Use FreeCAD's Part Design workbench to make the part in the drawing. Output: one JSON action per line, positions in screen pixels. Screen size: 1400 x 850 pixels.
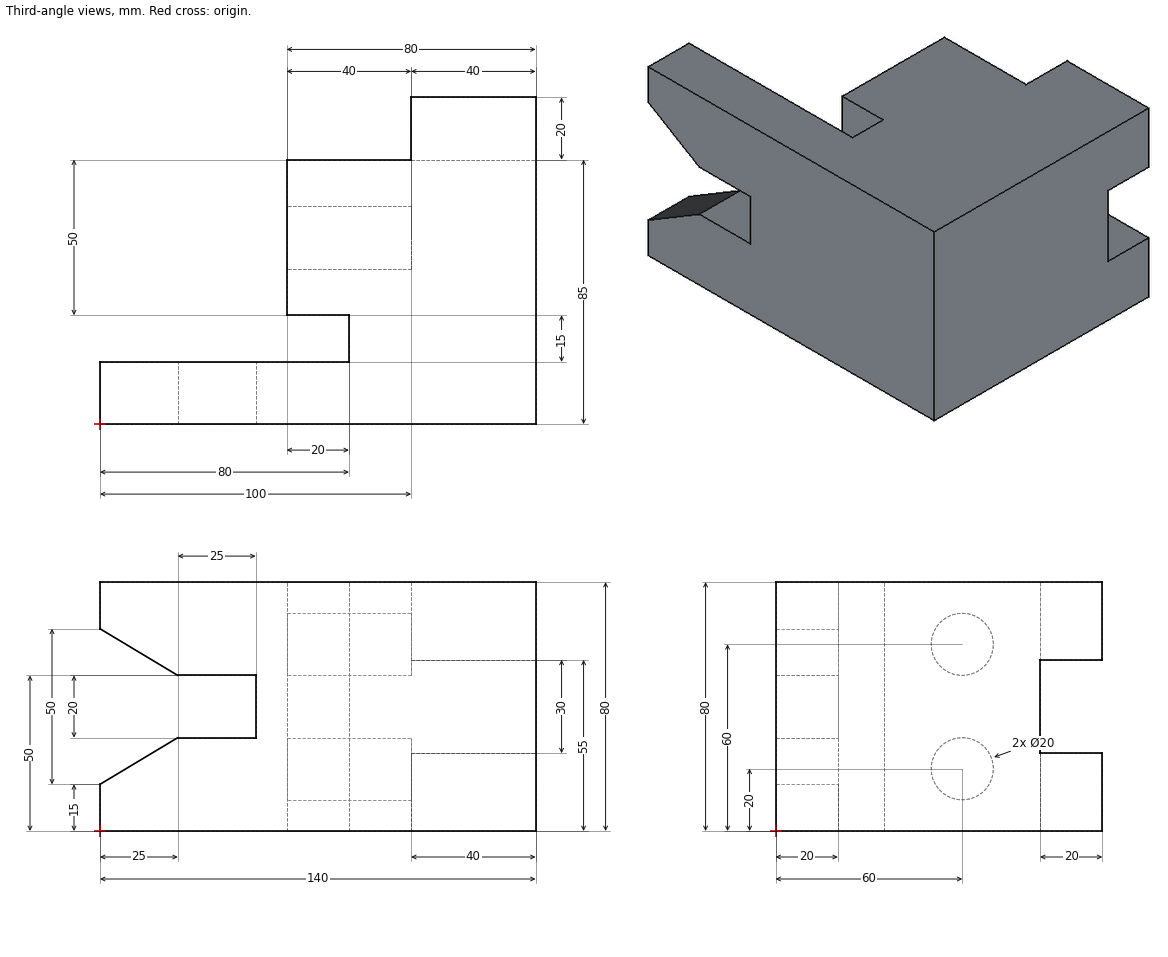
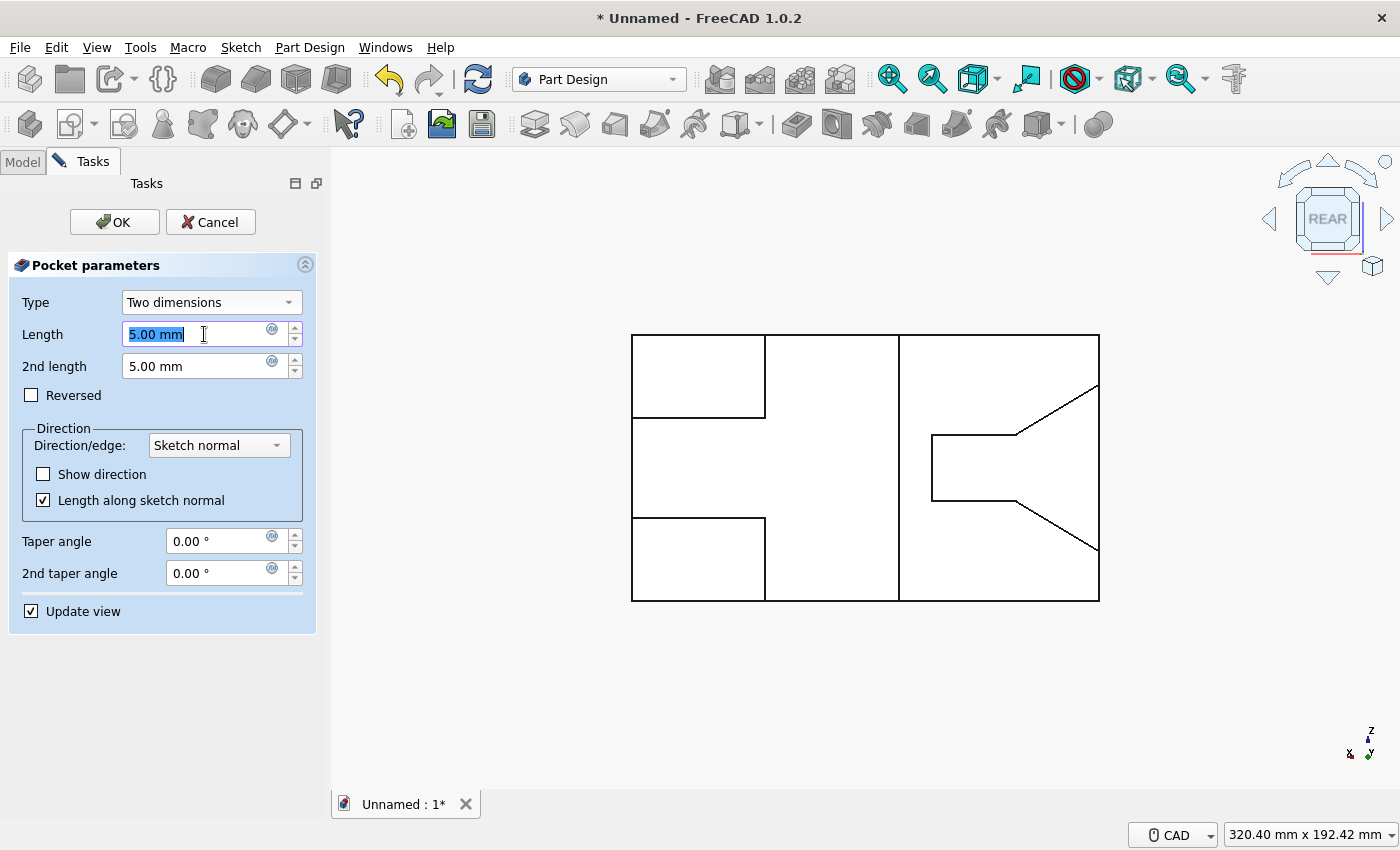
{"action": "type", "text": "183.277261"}
{"action": "key", "text": "Tab"}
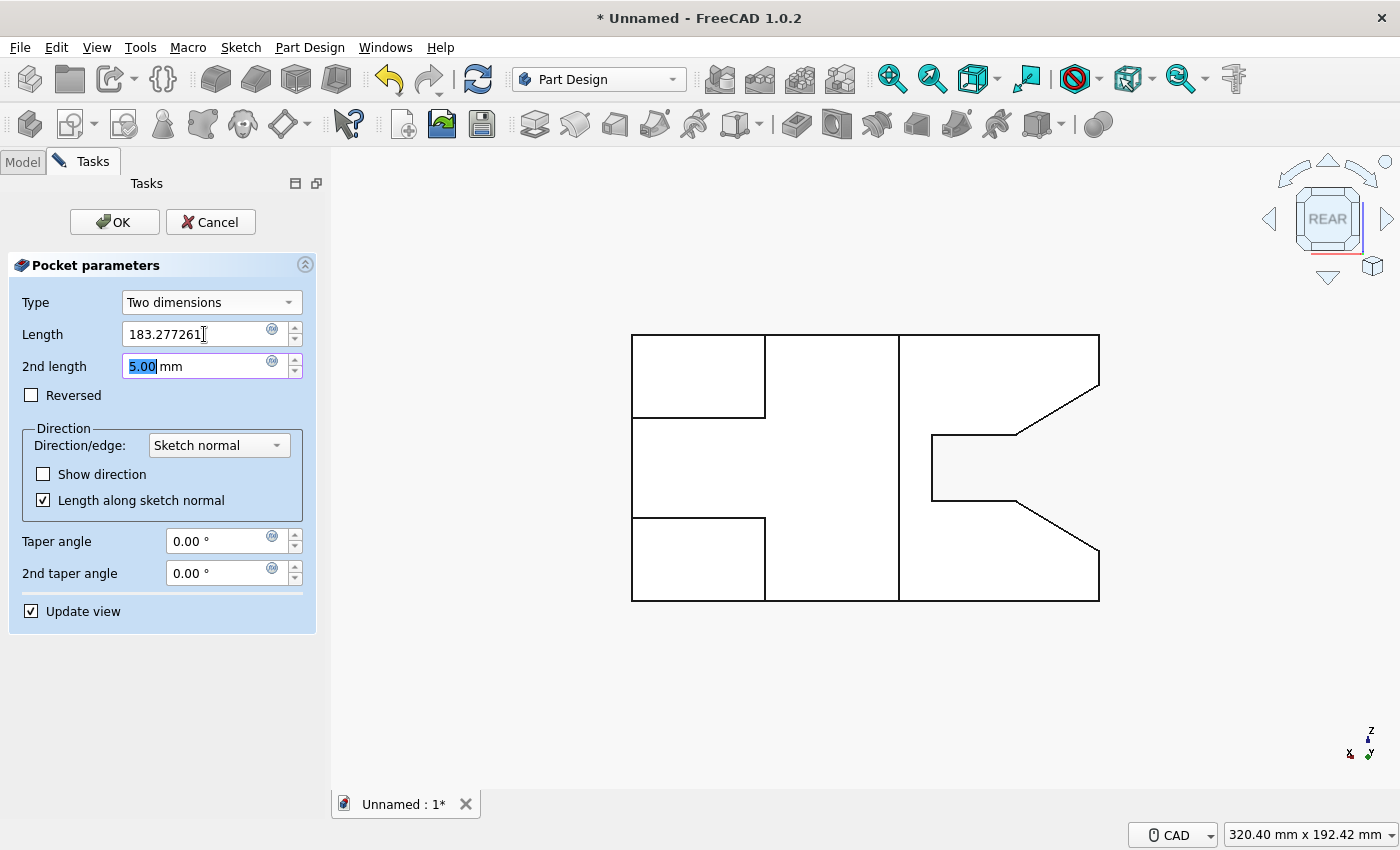
{"action": "type", "text": "20"}
{"action": "key", "text": "Tab"}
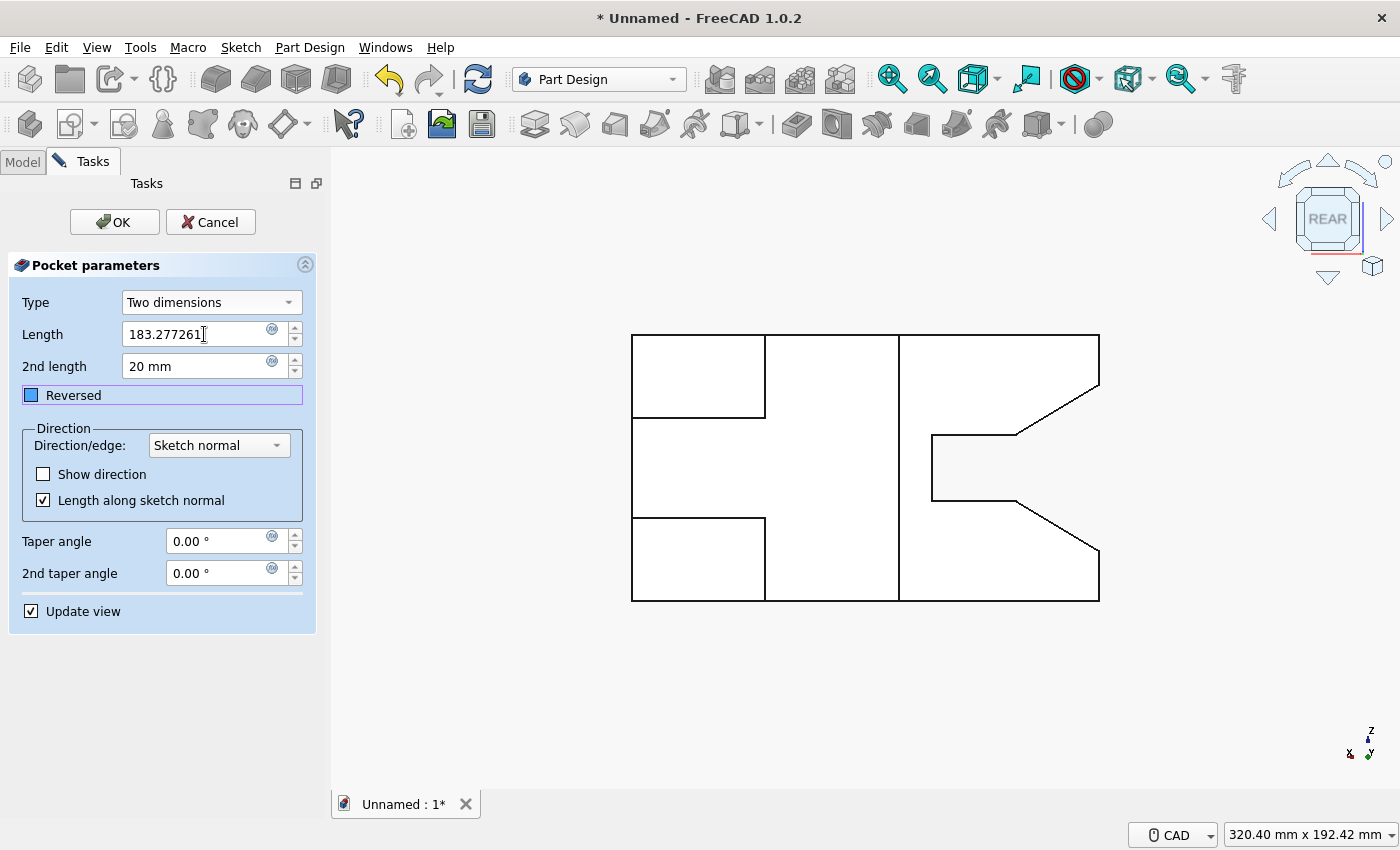
{"action": "left_click", "coordinate": [30, 395]}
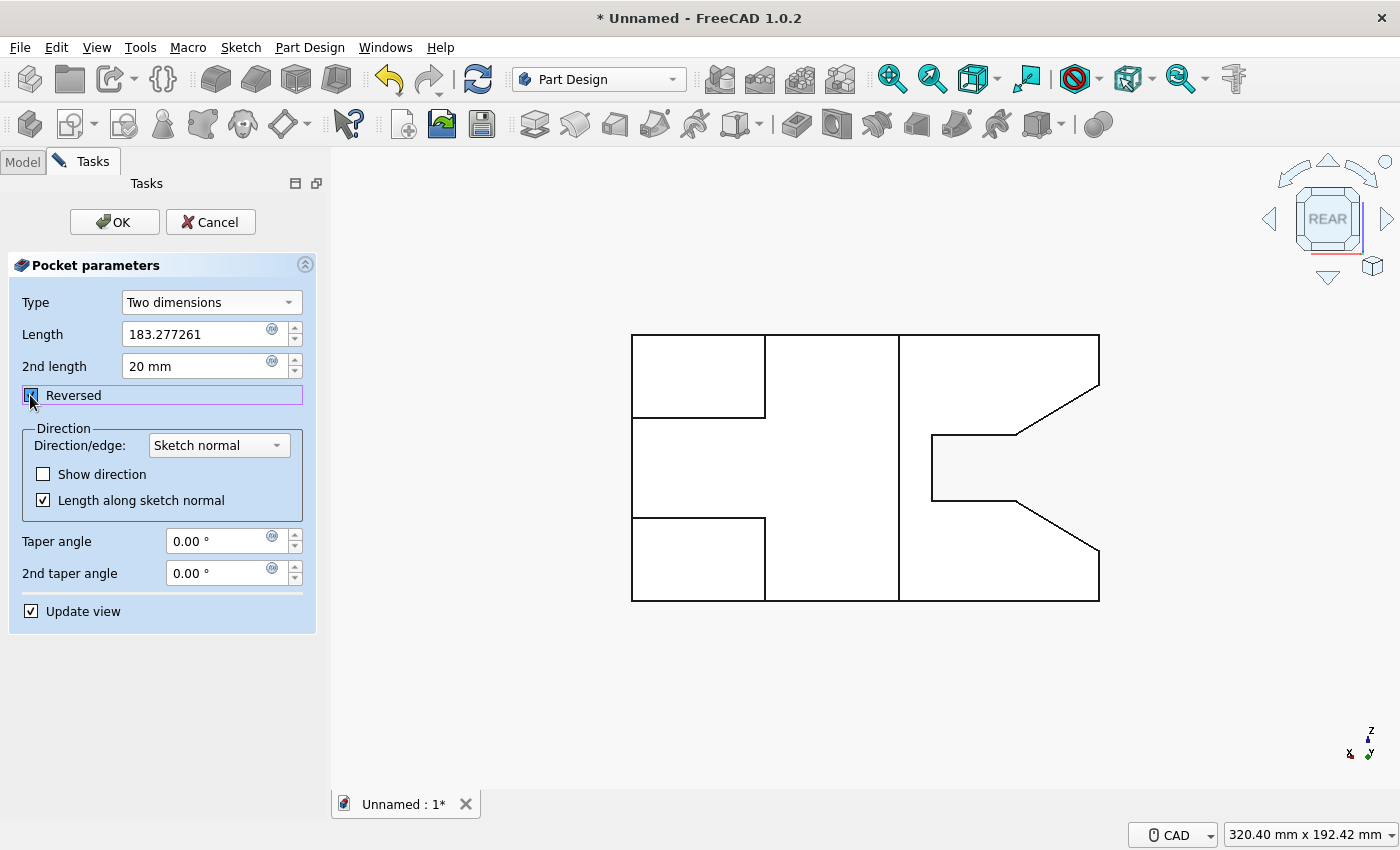
{"action": "left_click", "coordinate": [115, 222]}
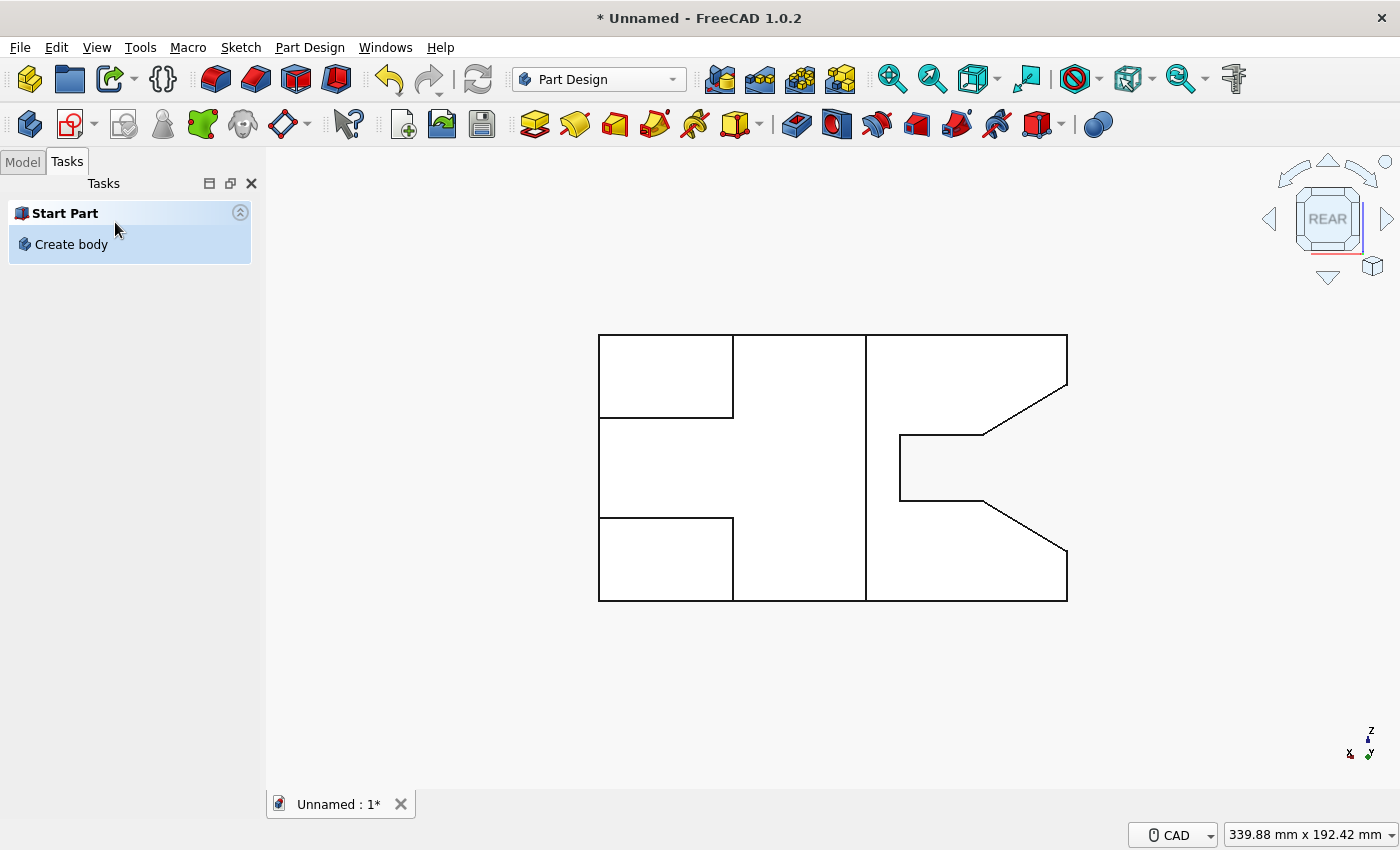
{"action": "key", "text": "v f"}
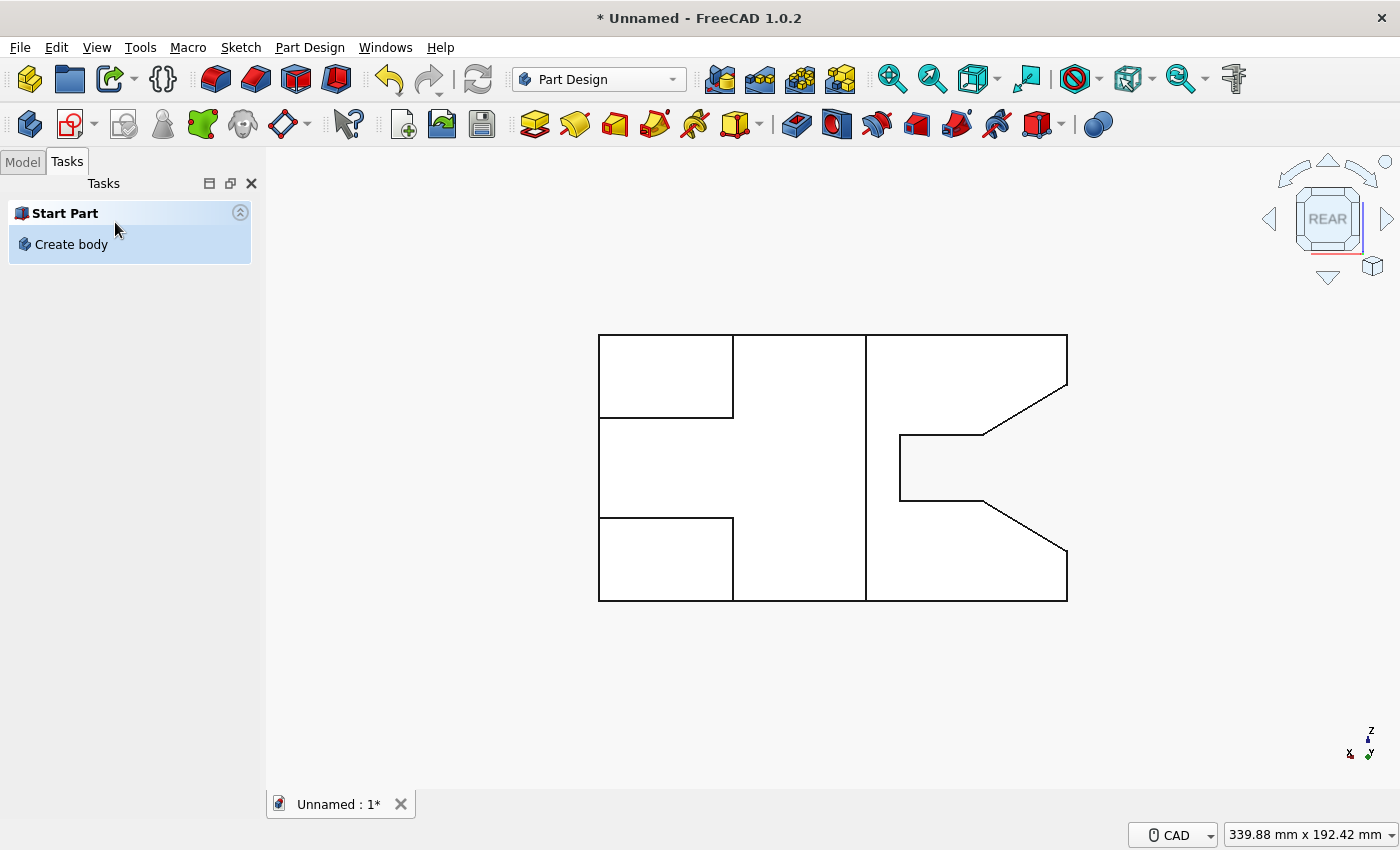
{"action": "key", "text": "6"}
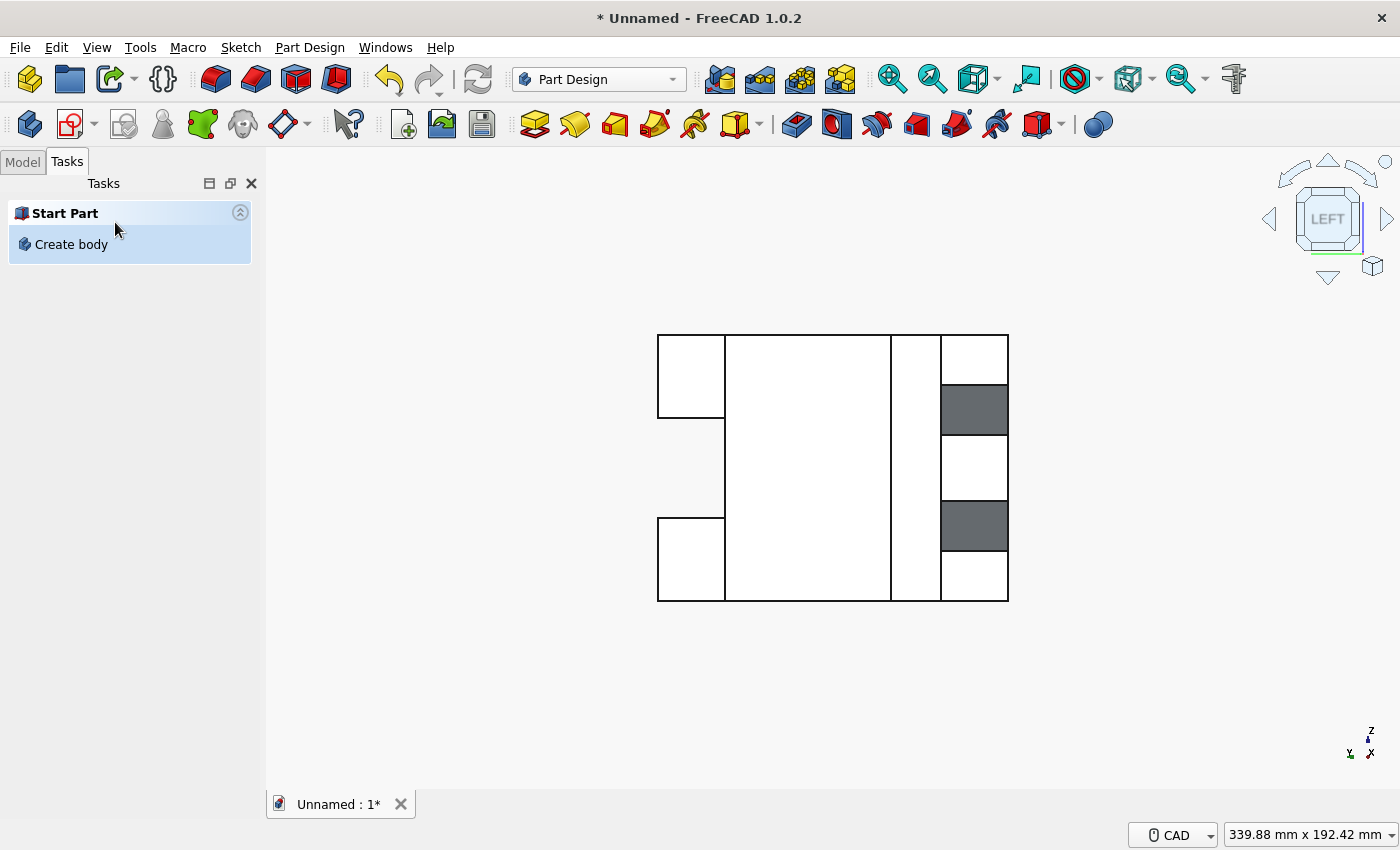
{"action": "key", "text": "v f"}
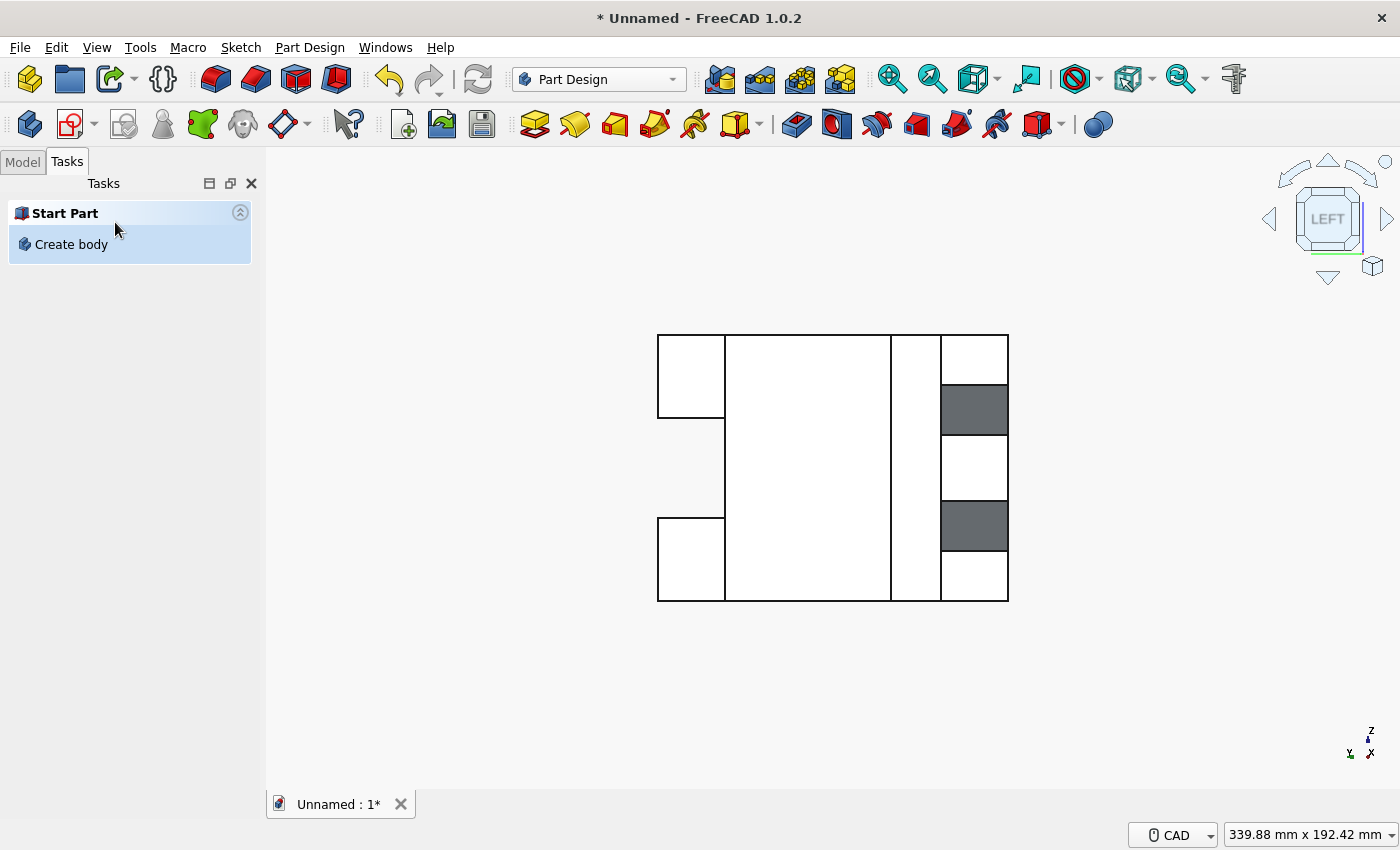
{"action": "left_click", "coordinate": [808, 429]}